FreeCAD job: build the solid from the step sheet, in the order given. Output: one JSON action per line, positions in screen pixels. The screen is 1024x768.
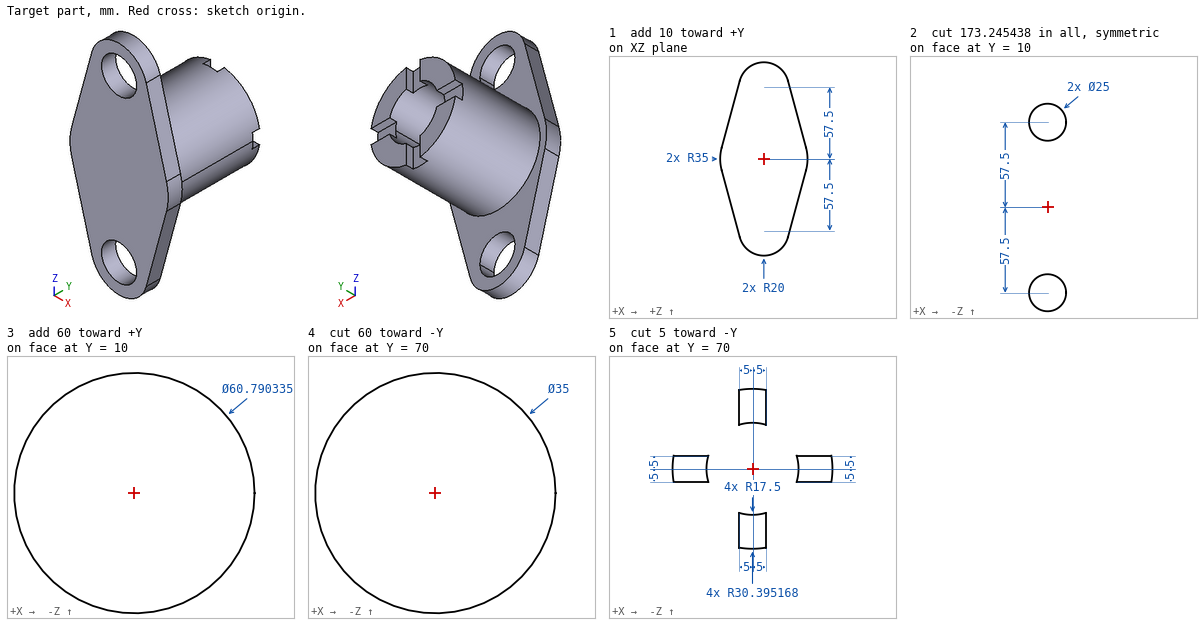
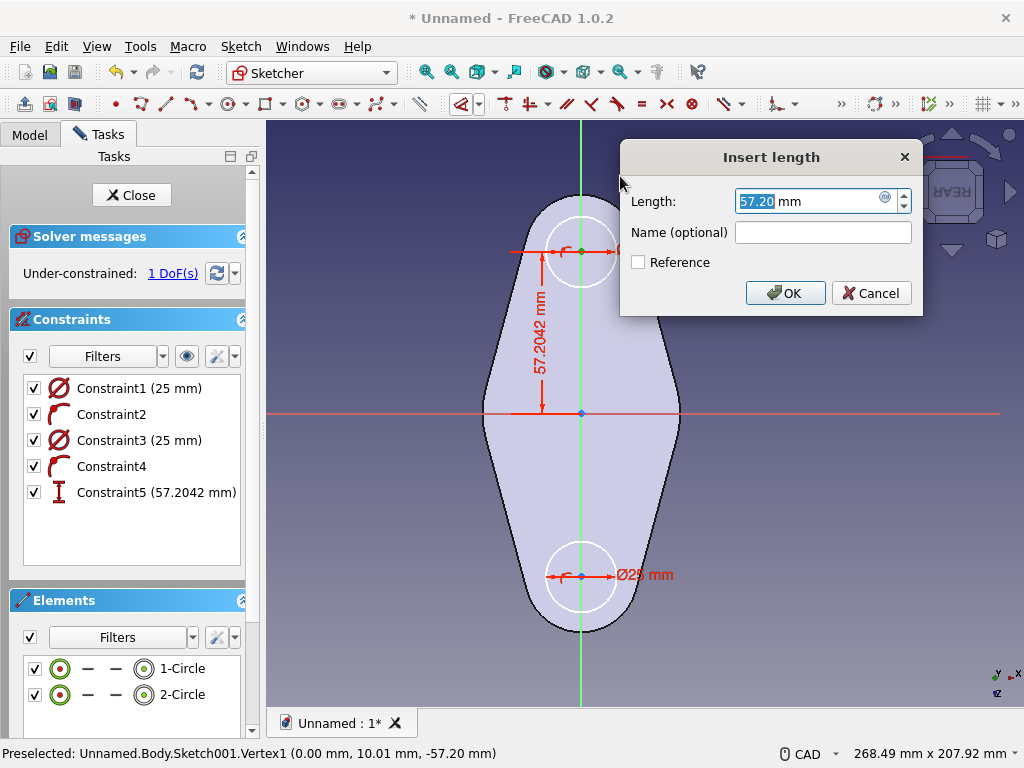
{"action": "type", "text": "57.5"}
{"action": "key", "text": "Return"}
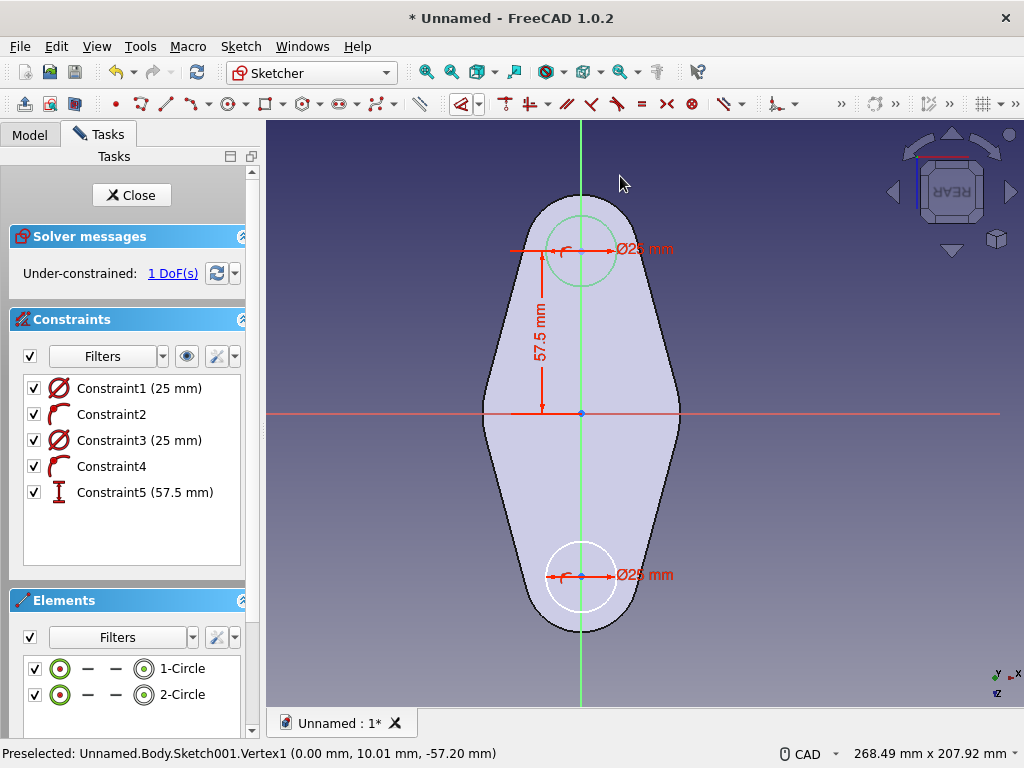
{"action": "left_click", "coordinate": [581, 577]}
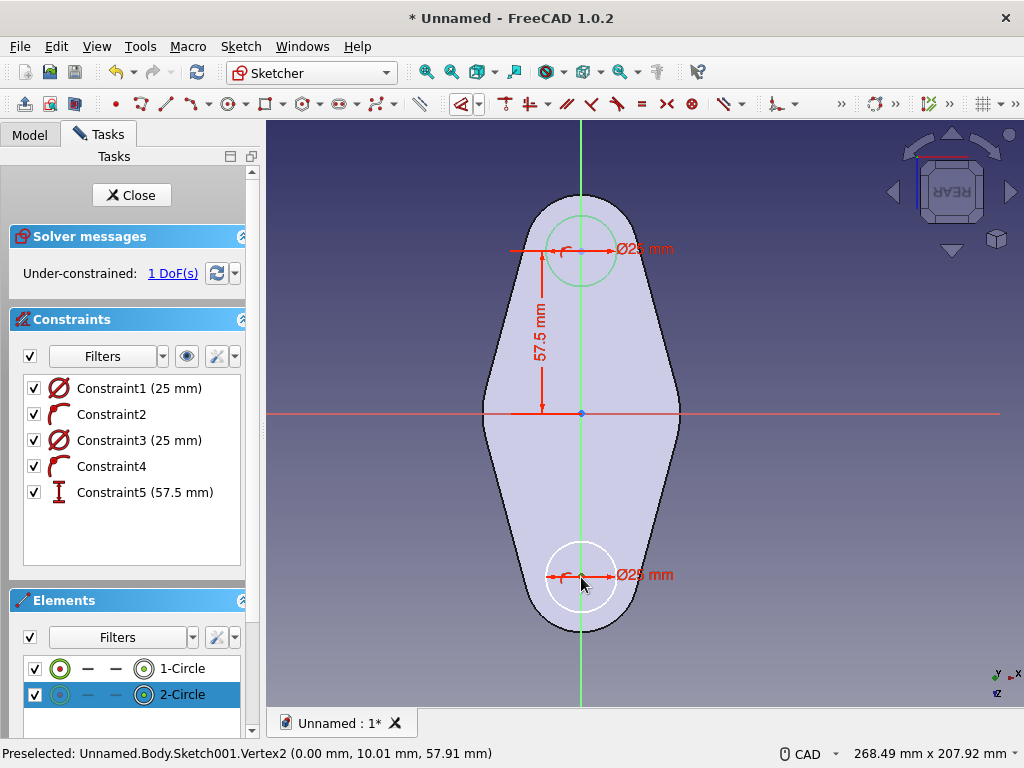
{"action": "left_click", "coordinate": [478, 104]}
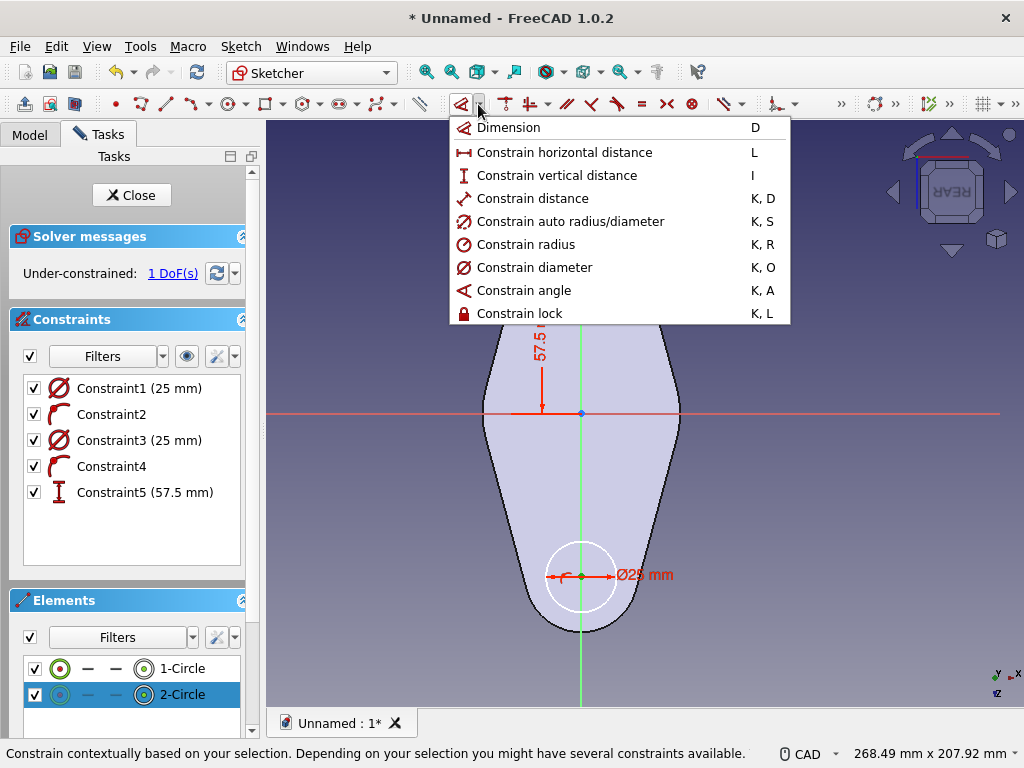
{"action": "left_click", "coordinate": [620, 176]}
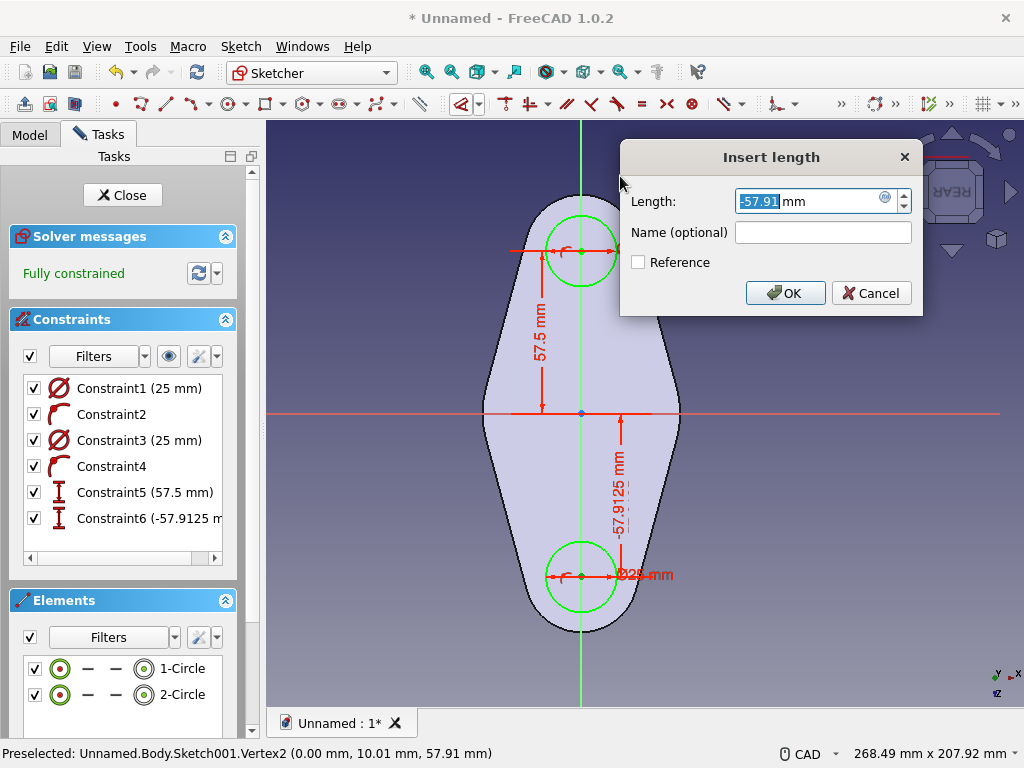
{"action": "type", "text": "-57.5"}
{"action": "key", "text": "Return"}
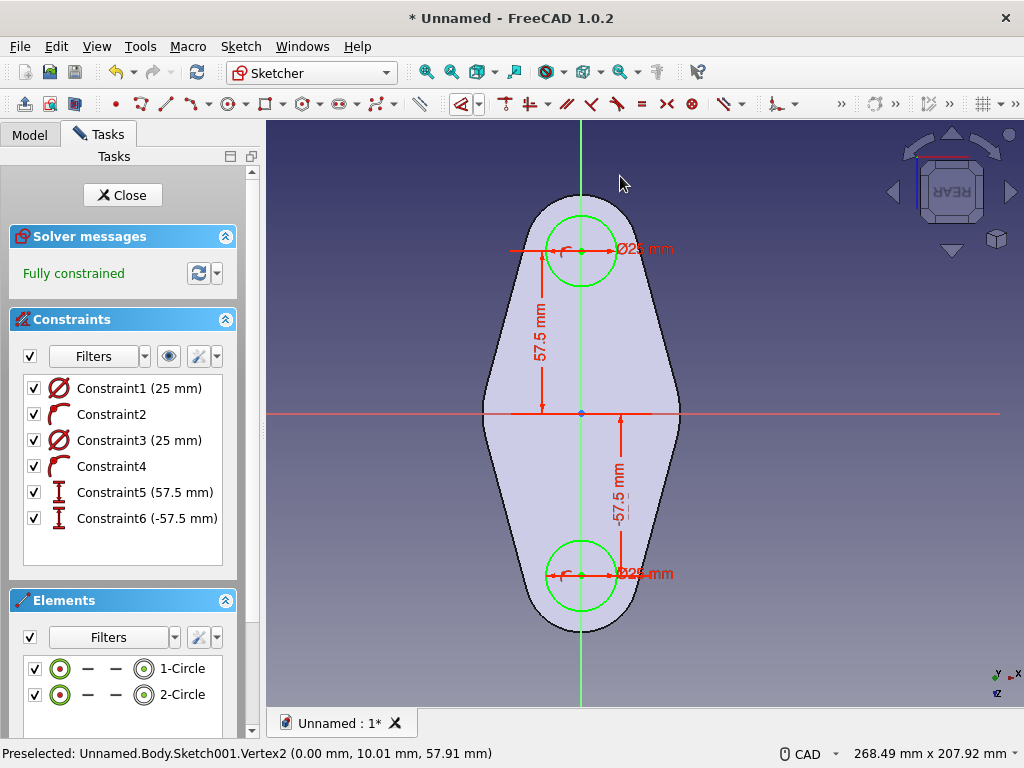
{"action": "left_click", "coordinate": [123, 195]}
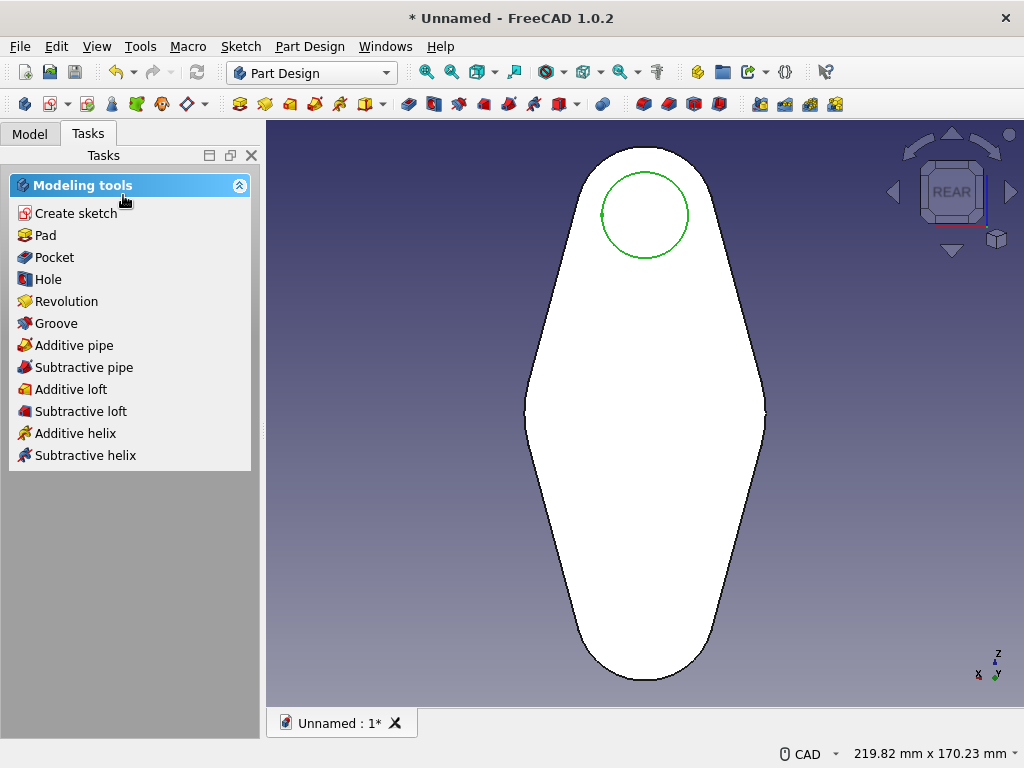
{"action": "left_click", "coordinate": [409, 104]}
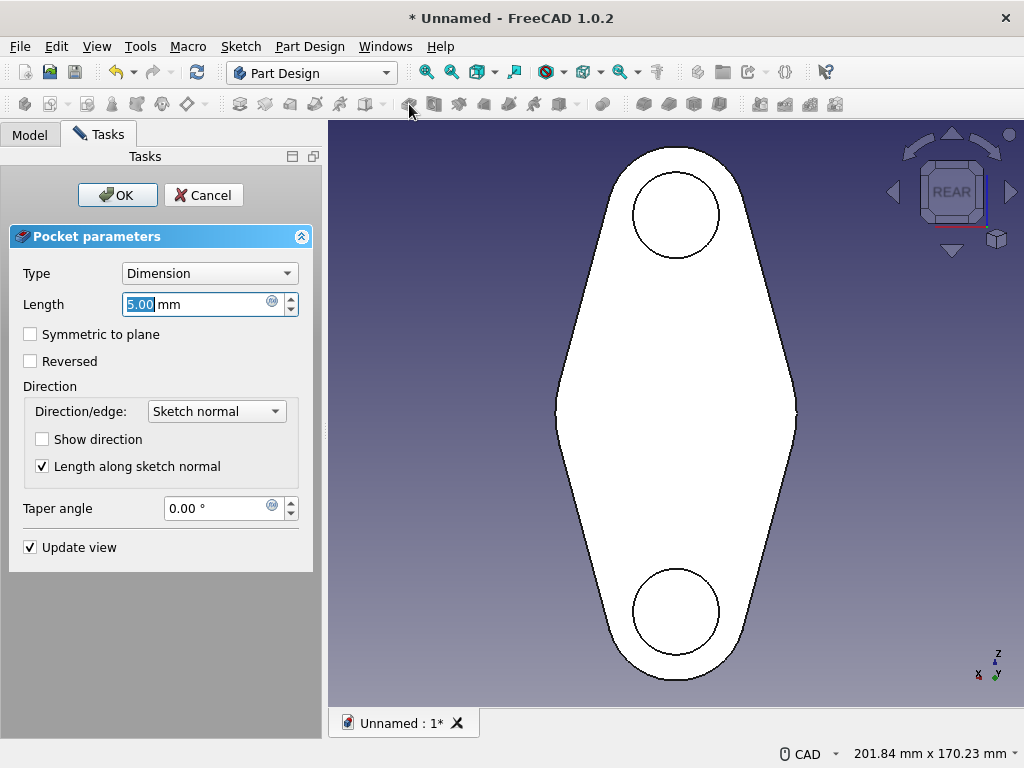
{"action": "type", "text": "173.245438"}
{"action": "key", "text": "Tab"}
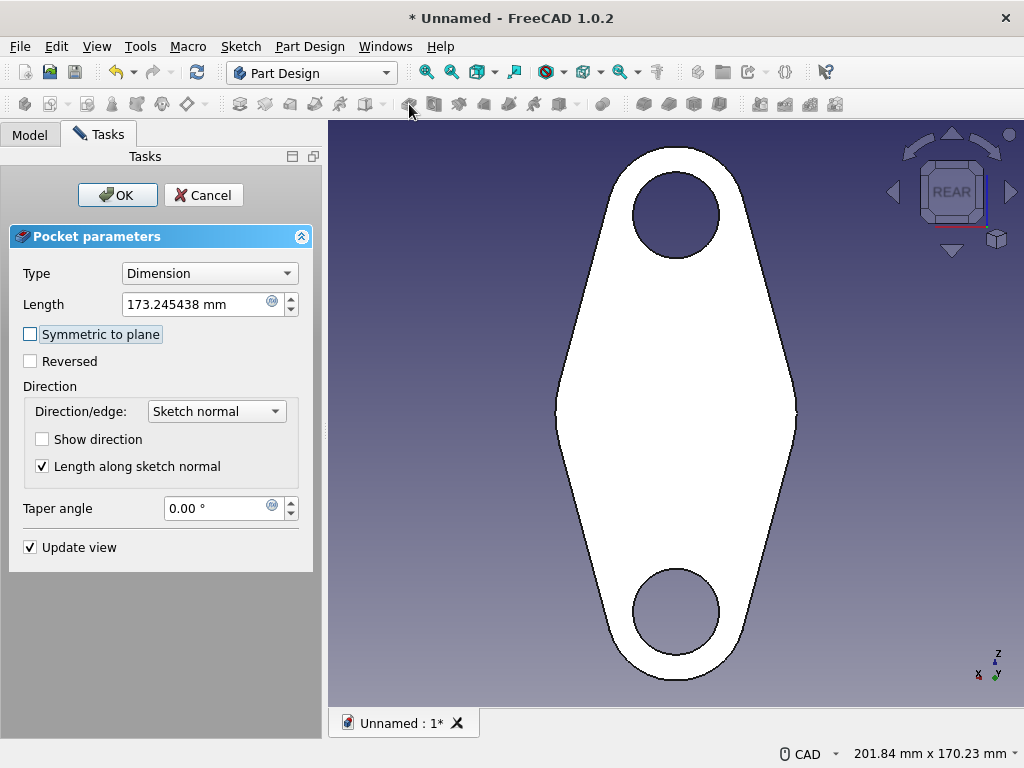
{"action": "left_click", "coordinate": [31, 334]}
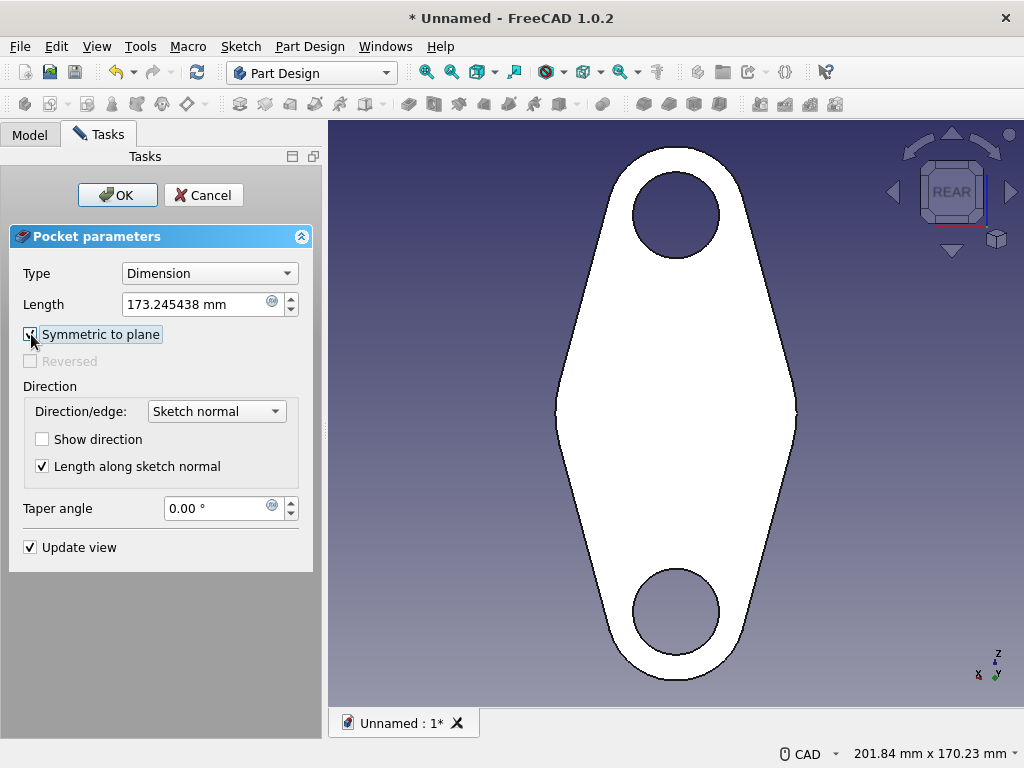
{"action": "left_click", "coordinate": [118, 195]}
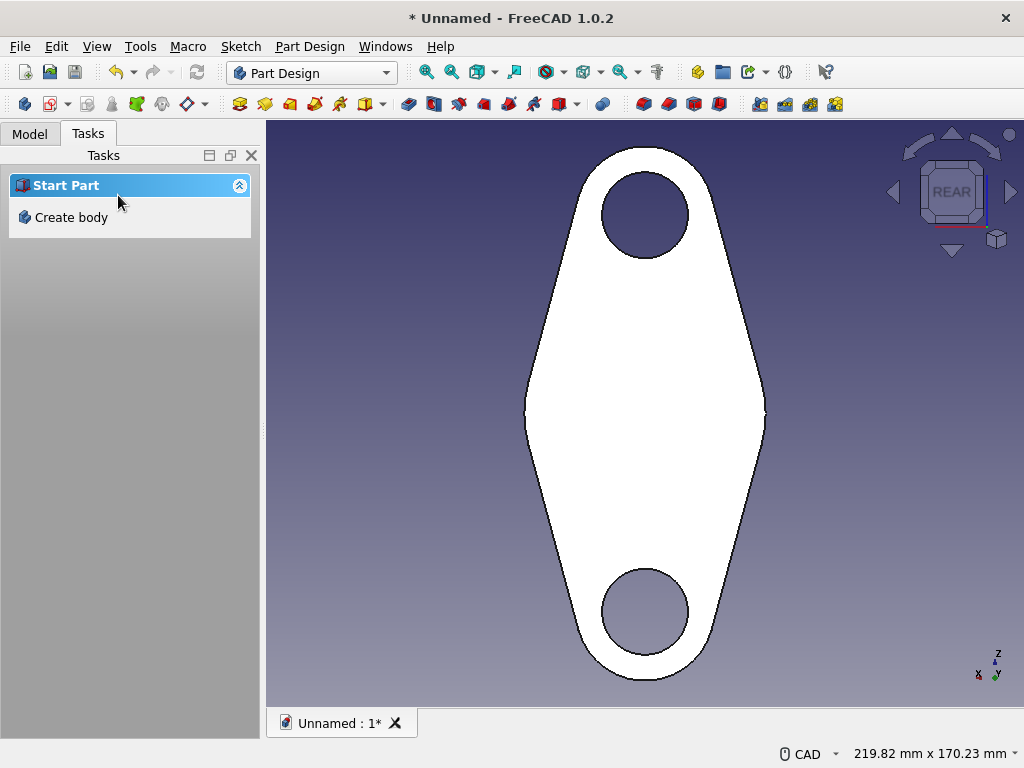
{"action": "left_click", "coordinate": [645, 412]}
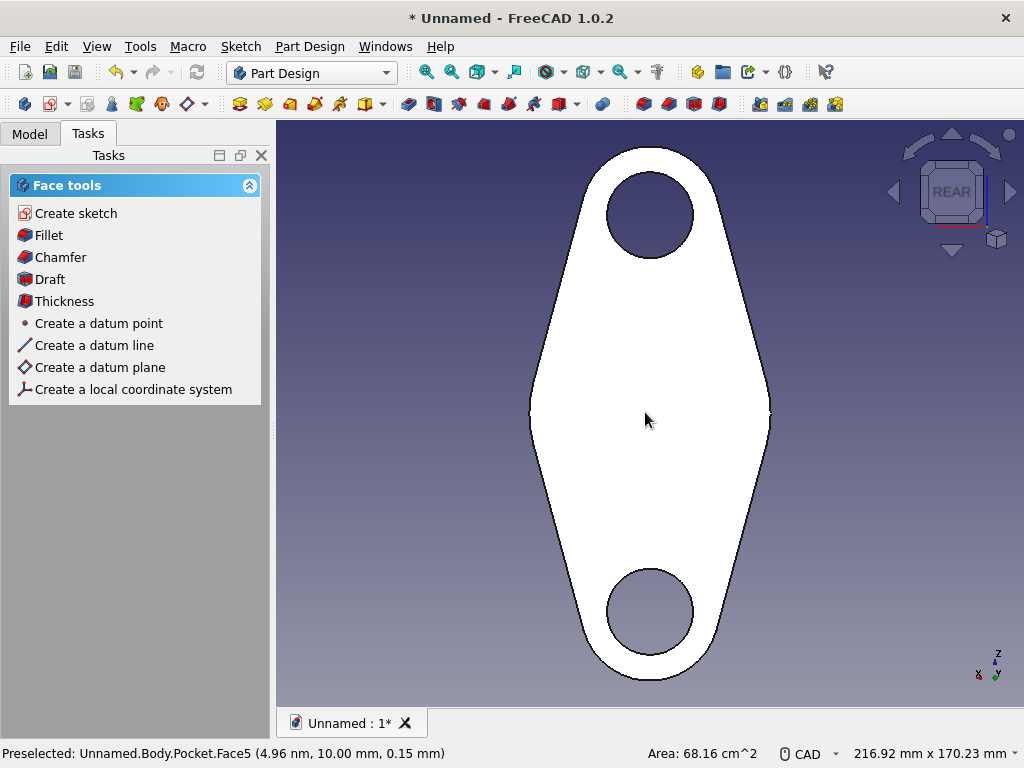
{"action": "left_click", "coordinate": [50, 104]}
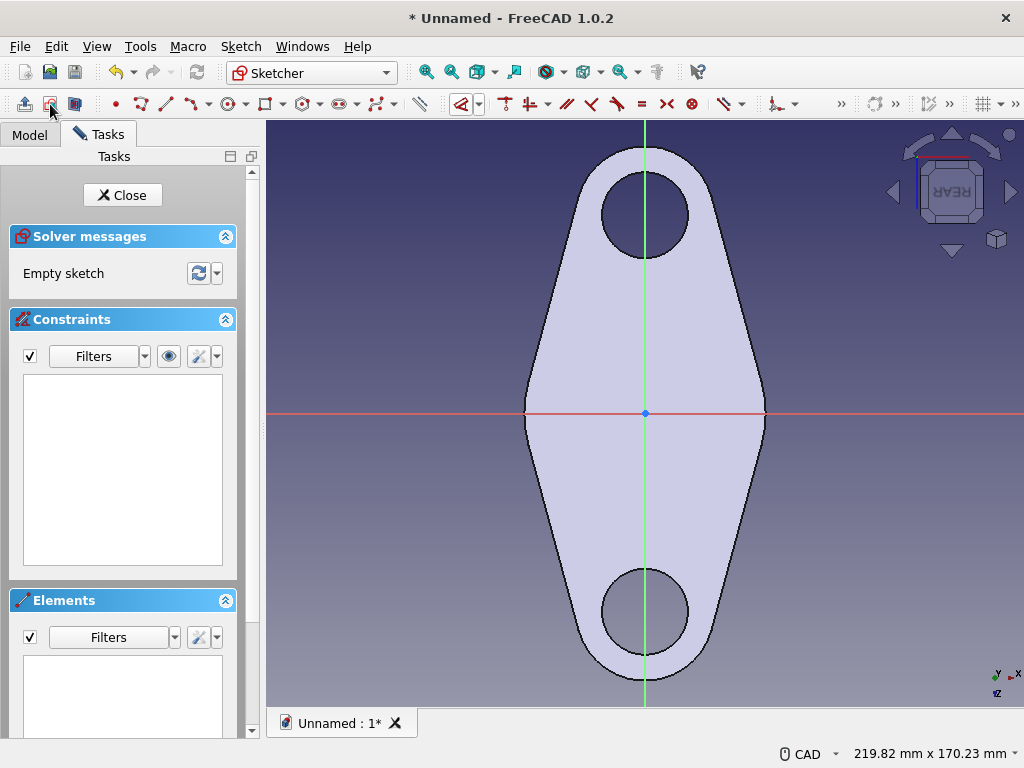
{"action": "scroll", "coordinate": [728, 413], "scroll_direction": "up", "scroll_amount": 3}